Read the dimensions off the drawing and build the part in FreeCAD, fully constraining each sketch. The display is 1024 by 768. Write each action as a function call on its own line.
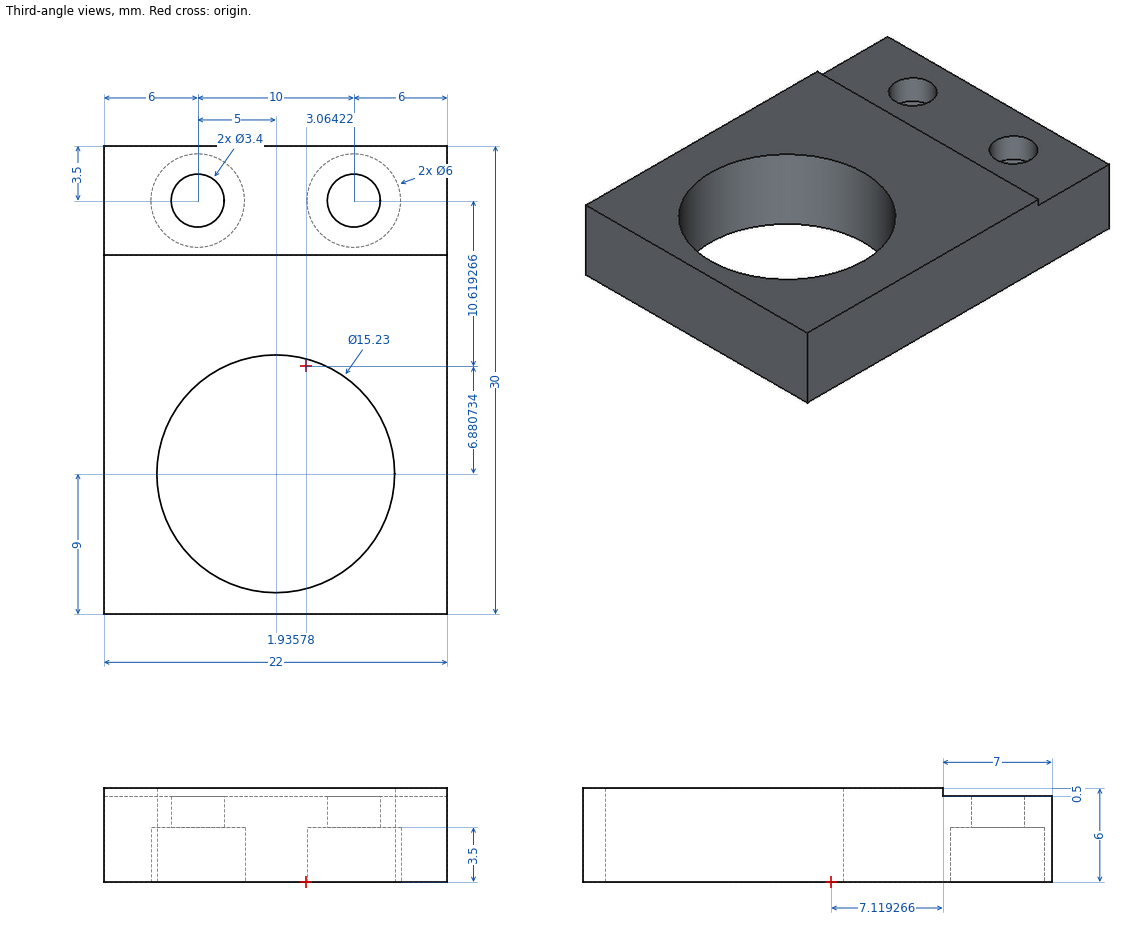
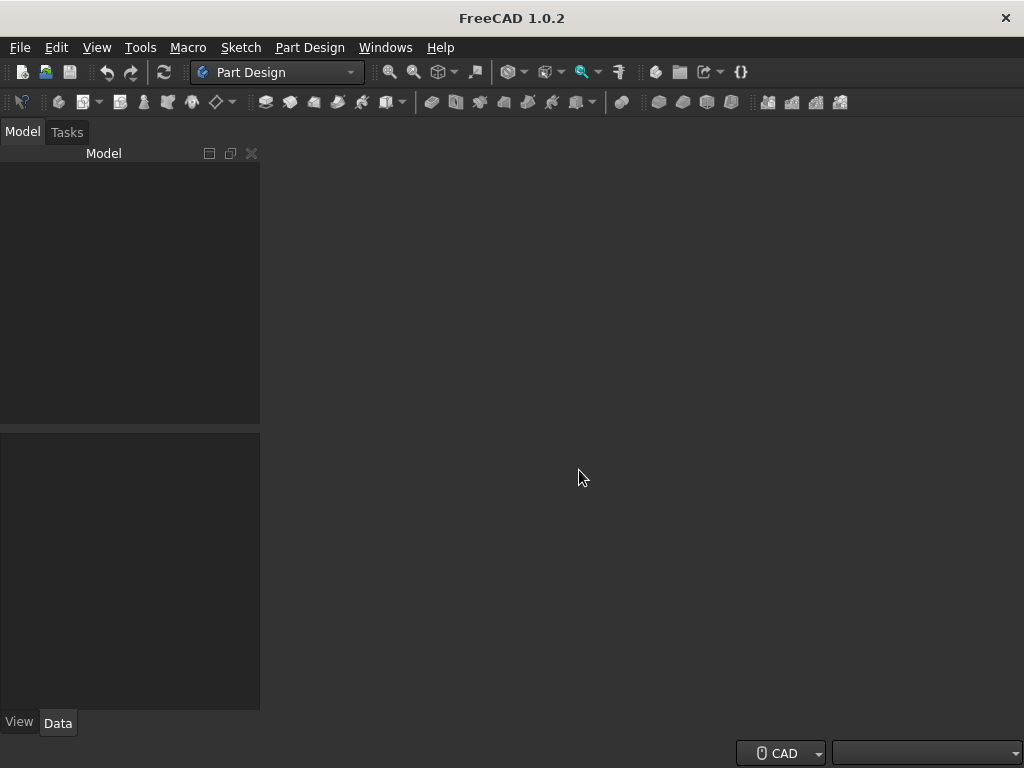
click(22, 72)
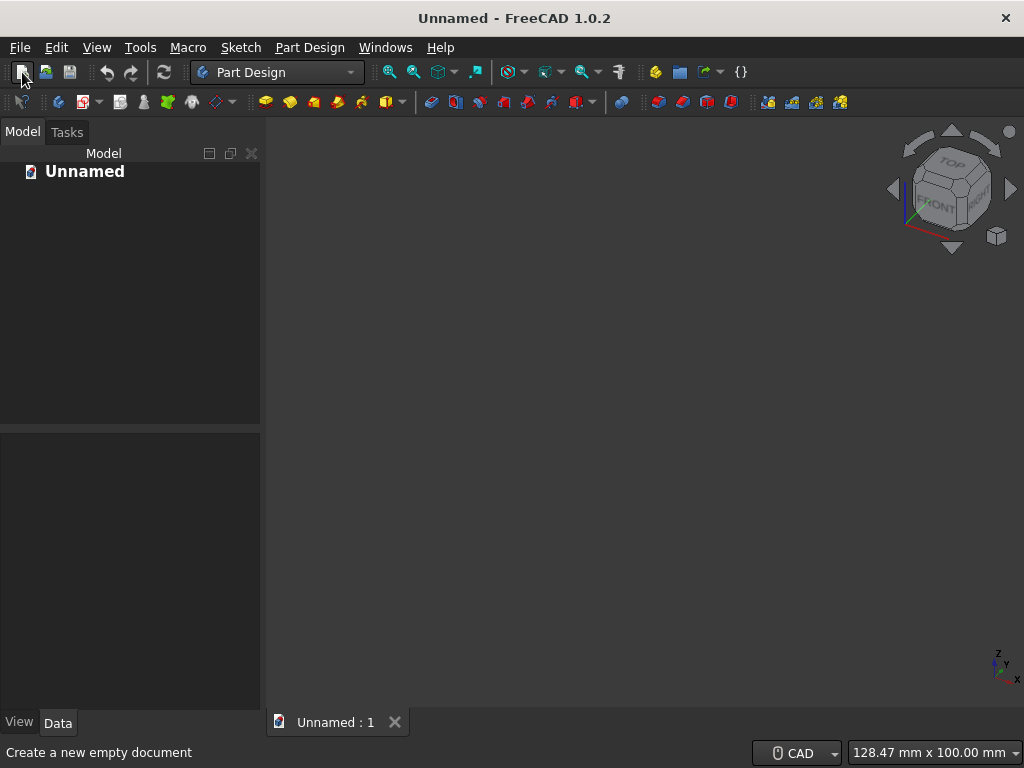
click(84, 102)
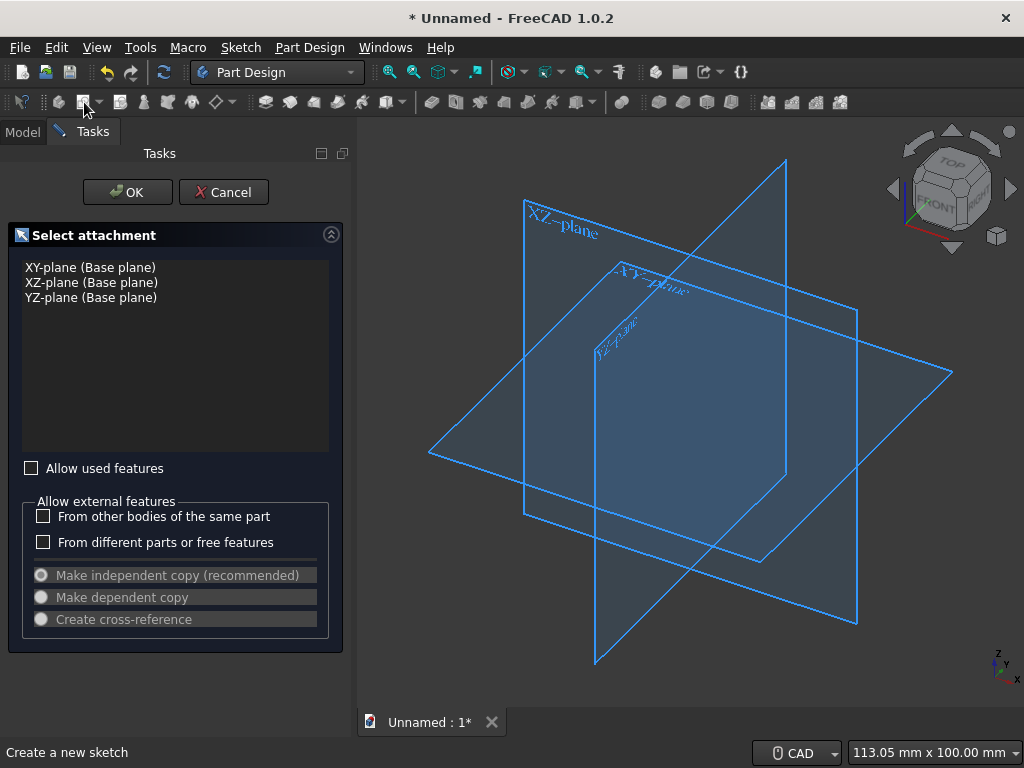
click(82, 268)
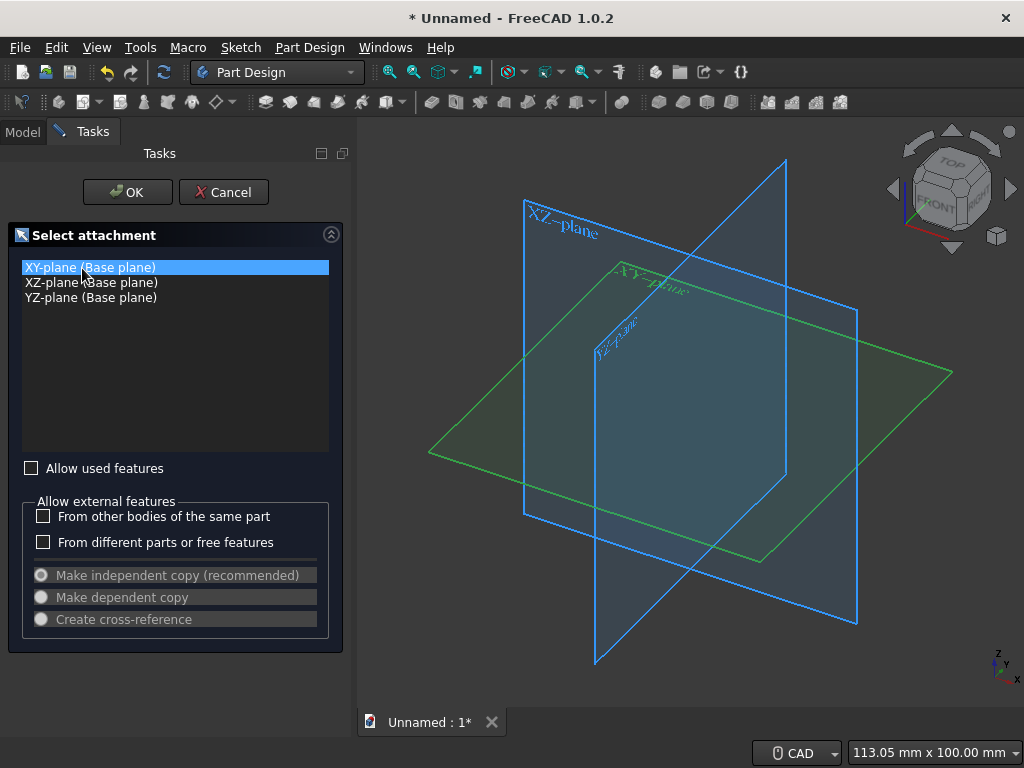
click(128, 192)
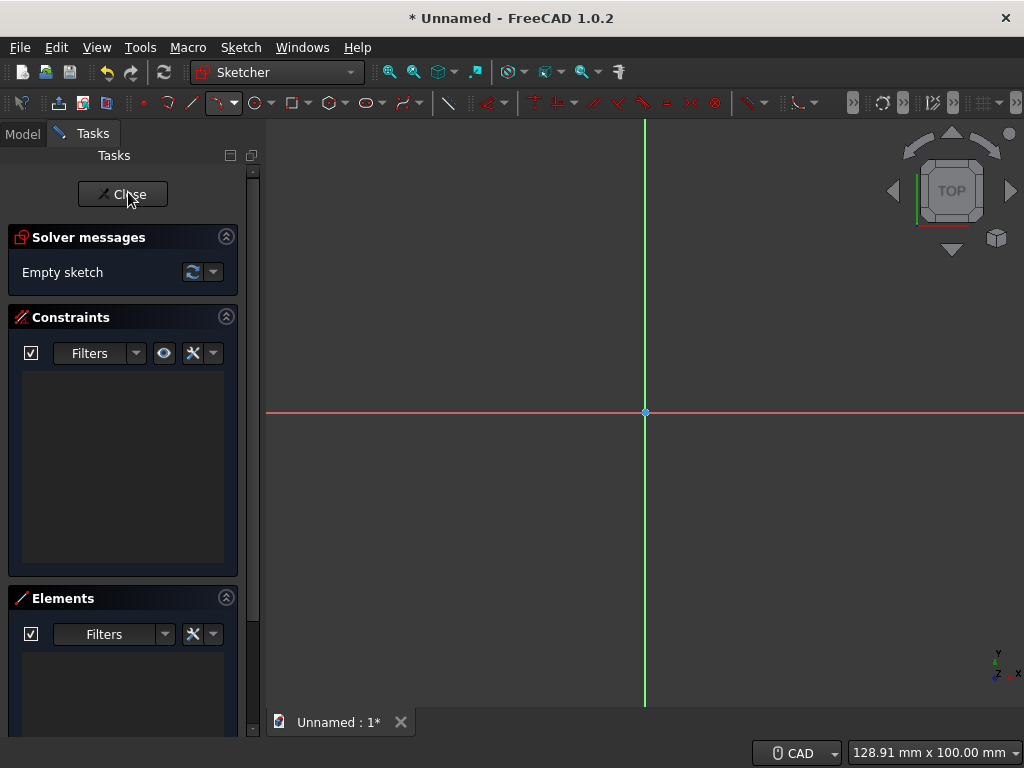
scroll(680, 422, up, 4)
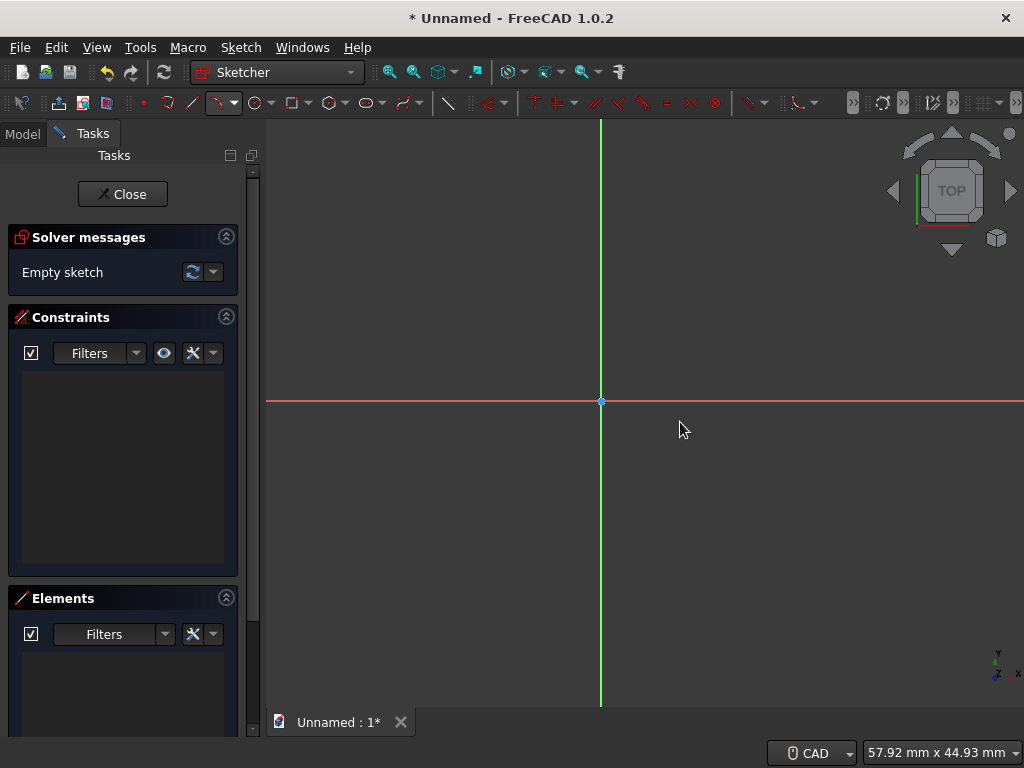
click(292, 104)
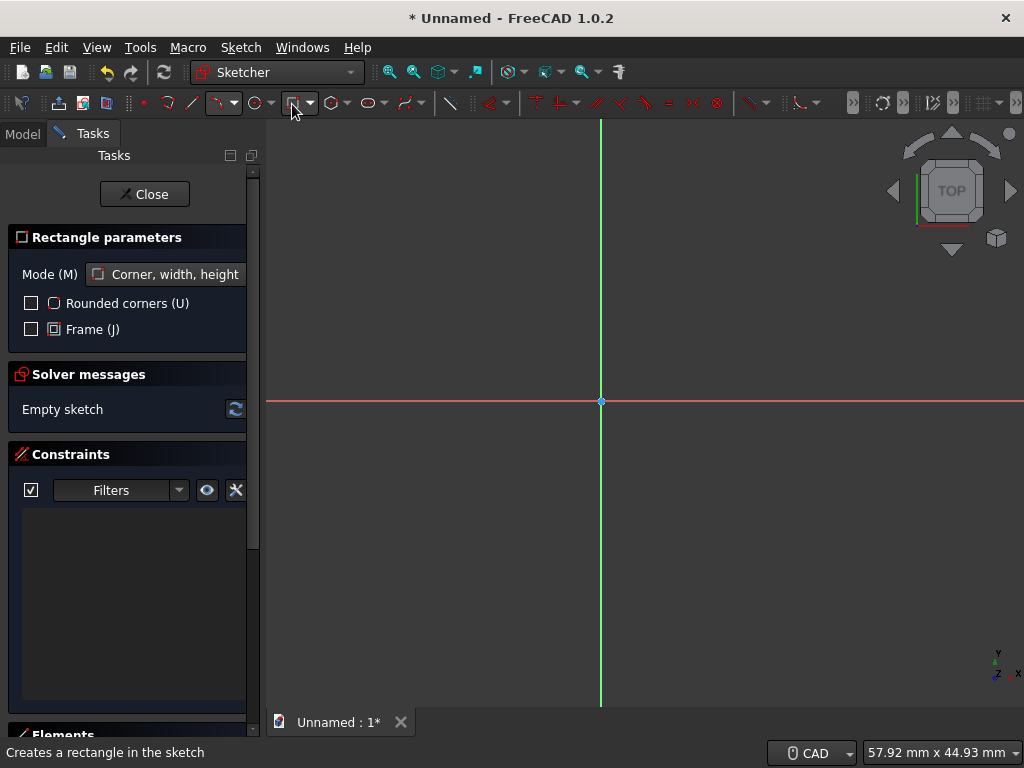
click(432, 217)
move(720, 609)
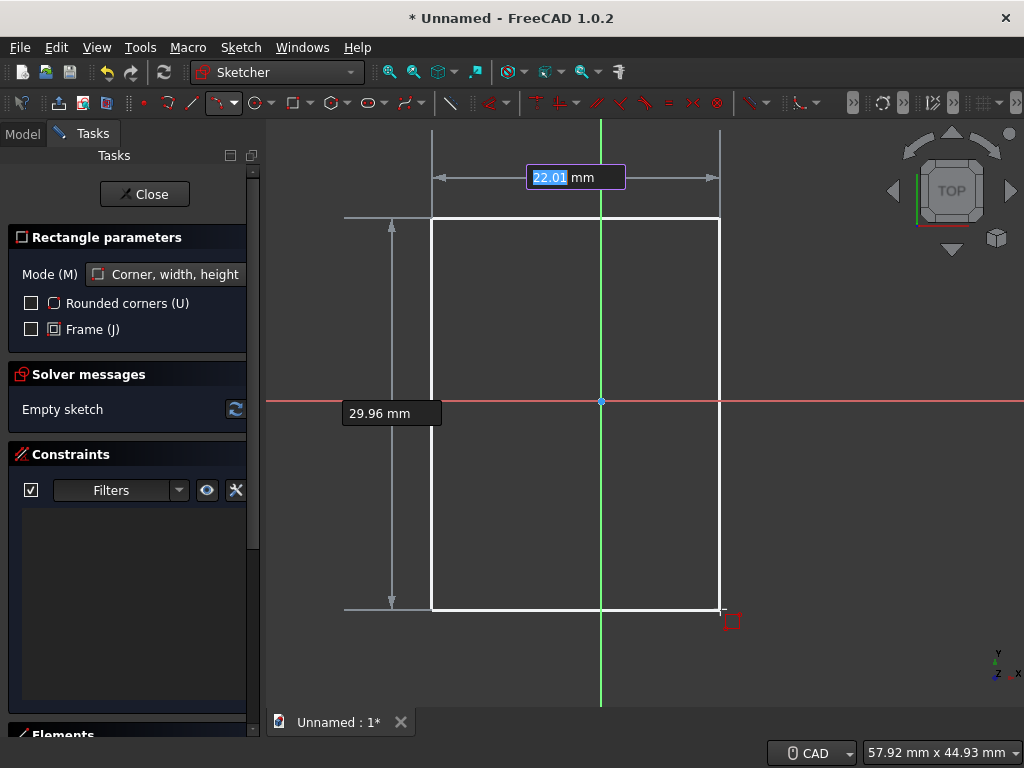
text(22)
key(Tab)
text(30)
key(Return)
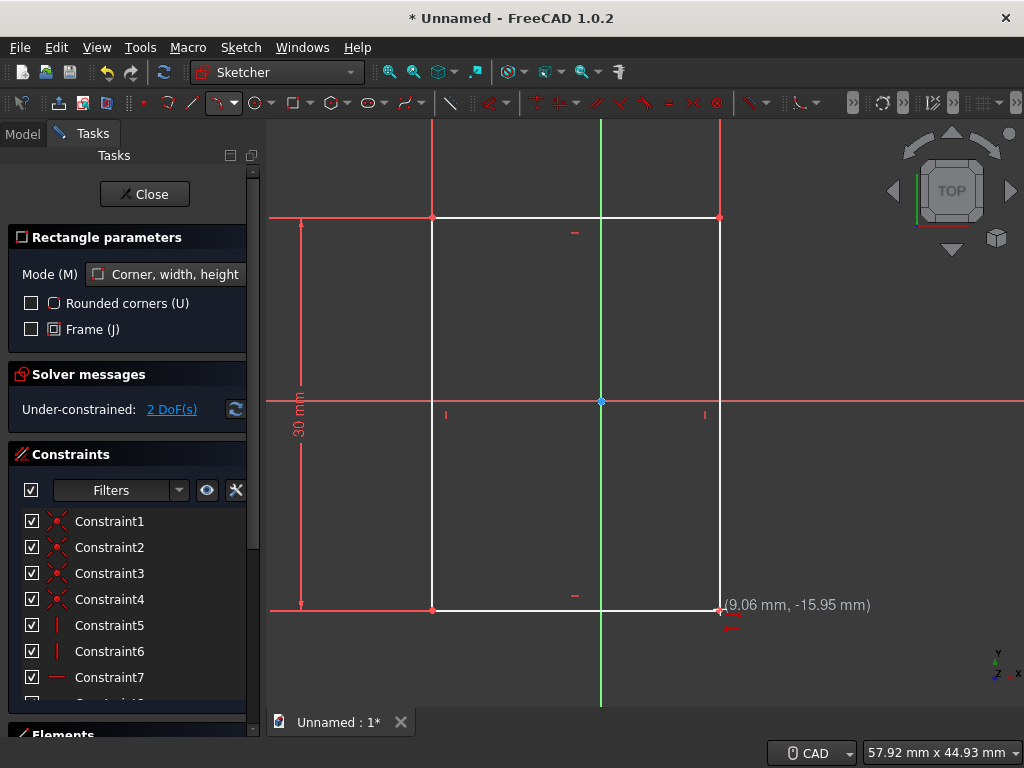
key(g)
key(c)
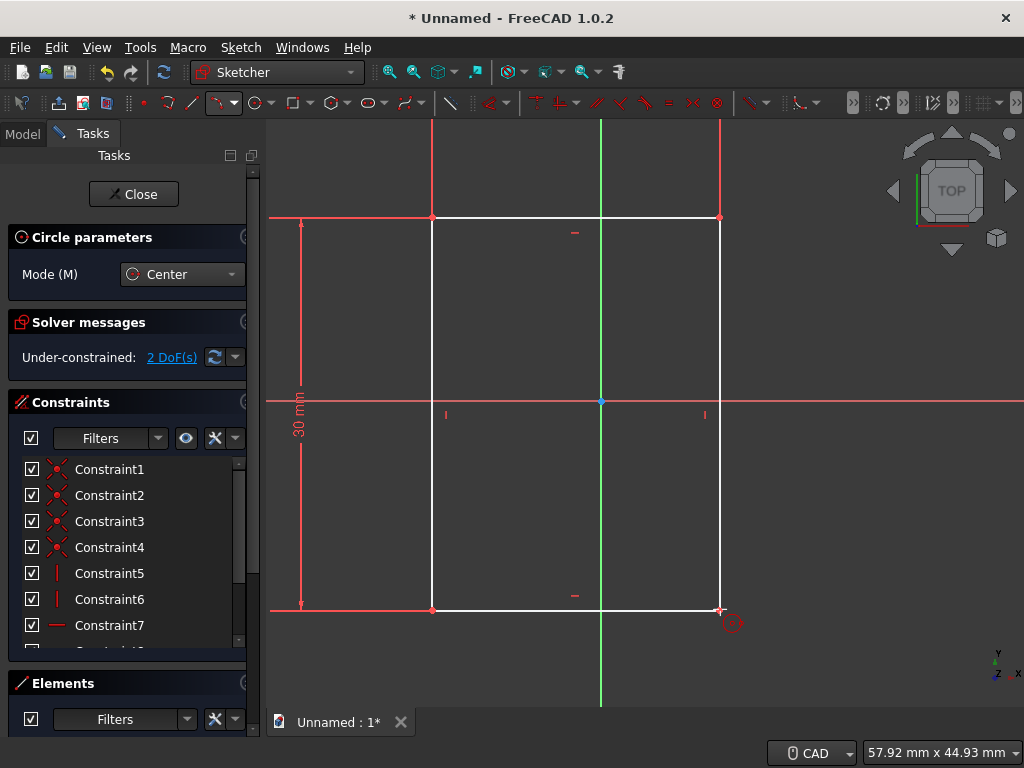
click(576, 491)
move(647, 421)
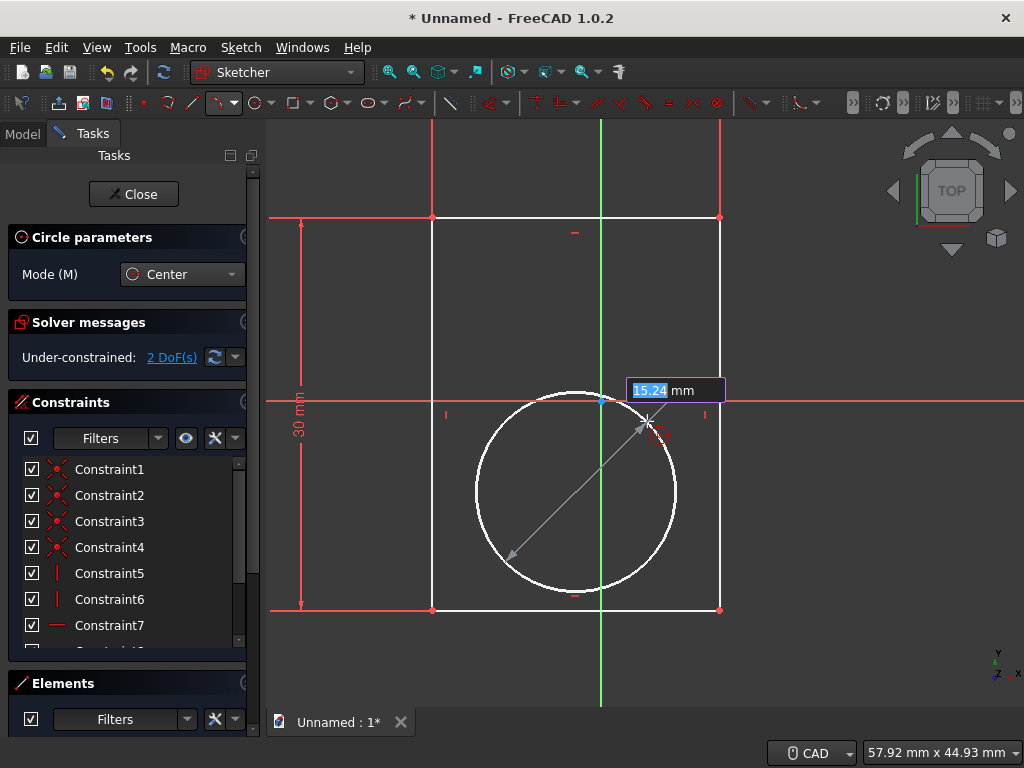
text(15.23)
key(Return)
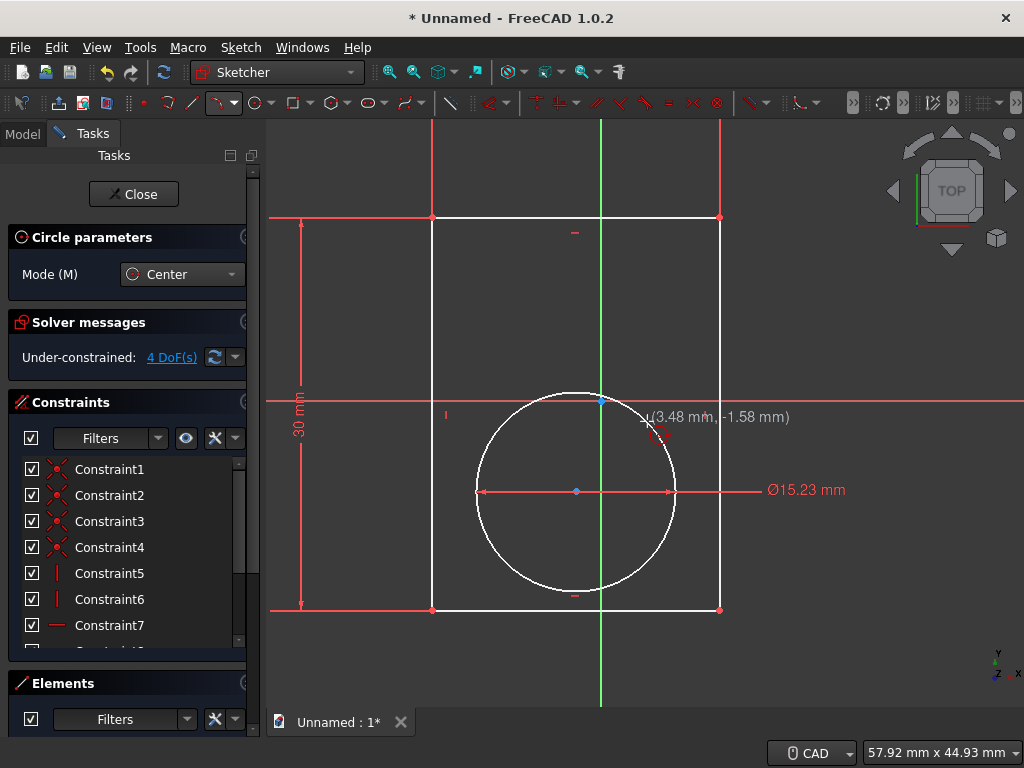
click(511, 262)
move(526, 247)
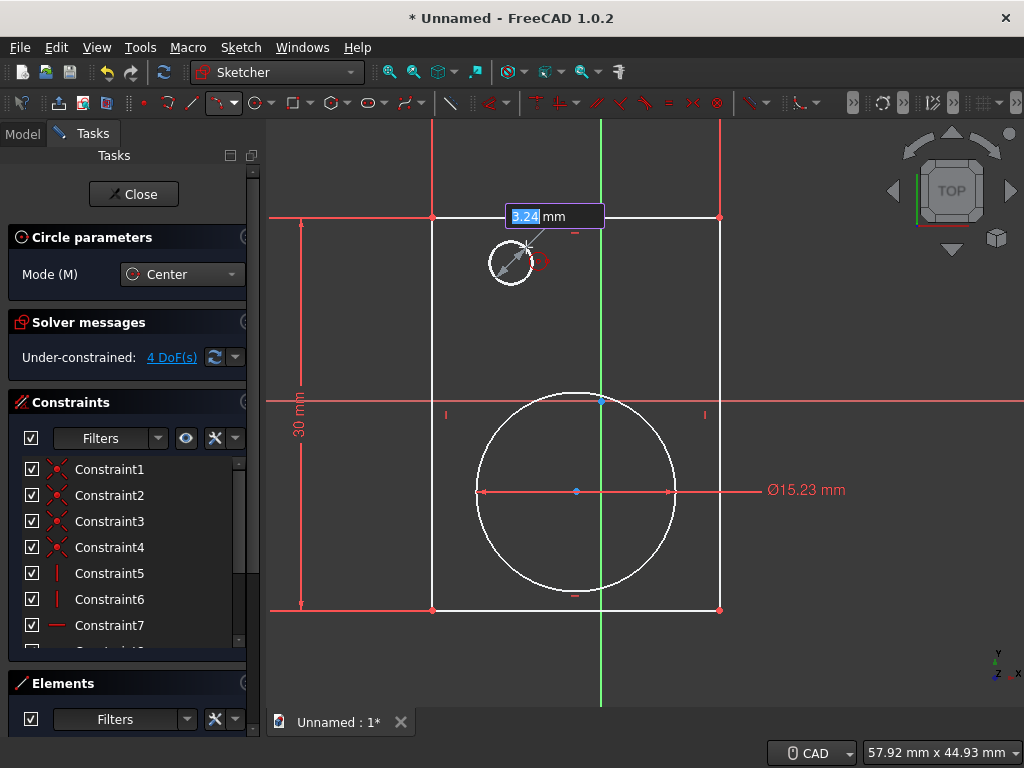
text(3.4)
key(Return)